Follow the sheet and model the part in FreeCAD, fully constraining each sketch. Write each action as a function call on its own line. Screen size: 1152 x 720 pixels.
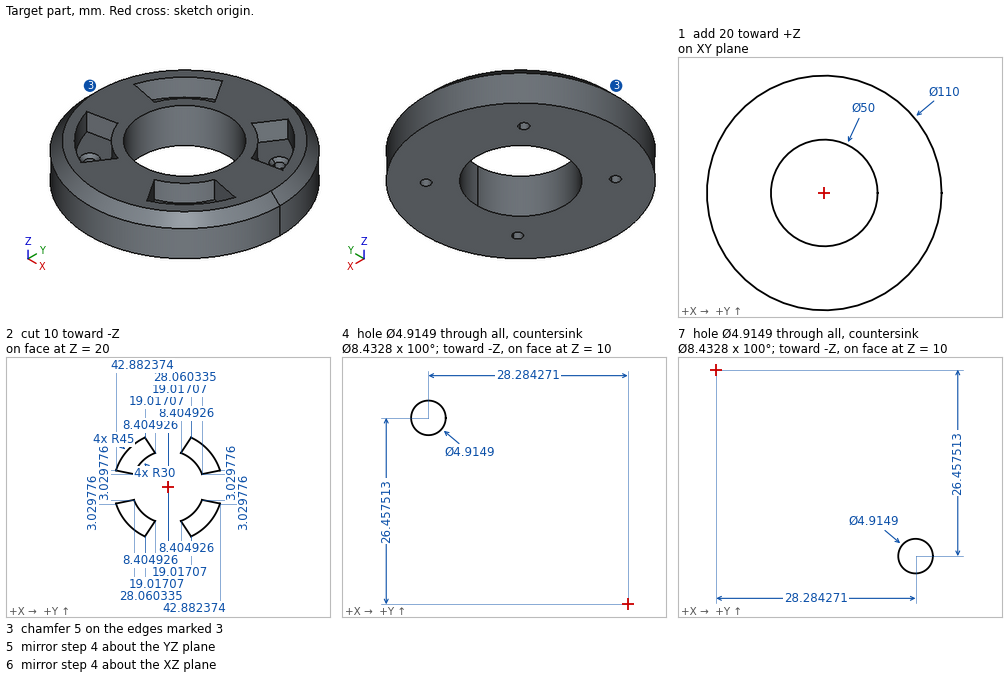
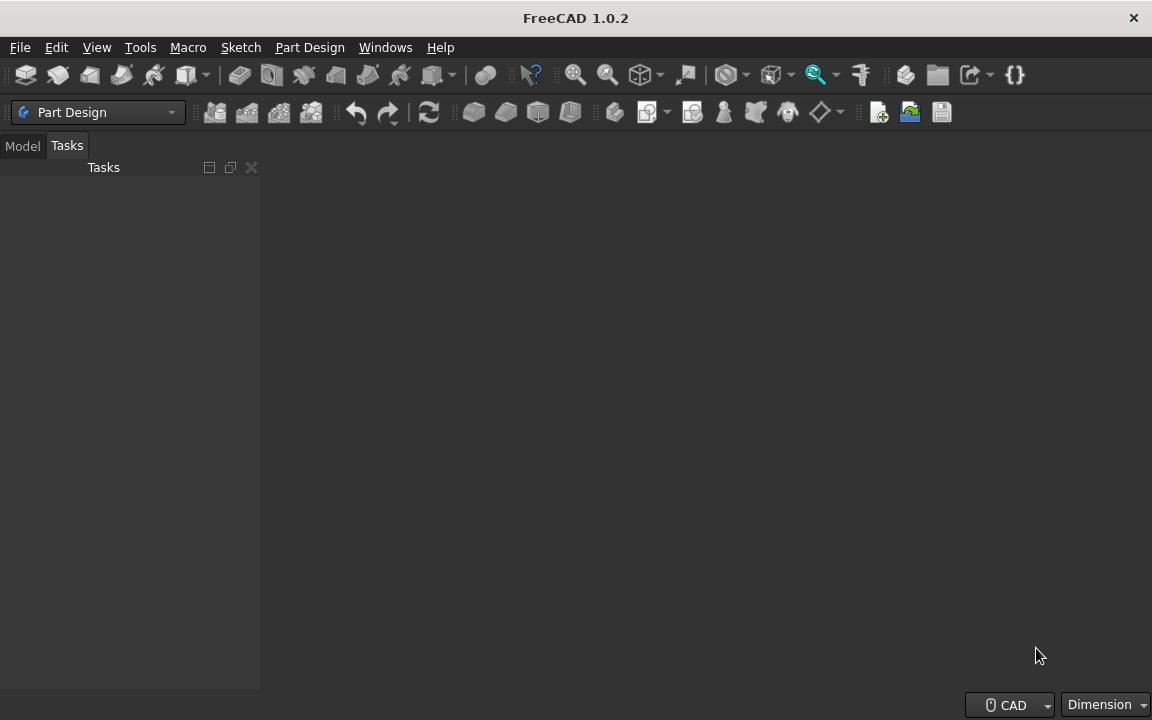
click(878, 112)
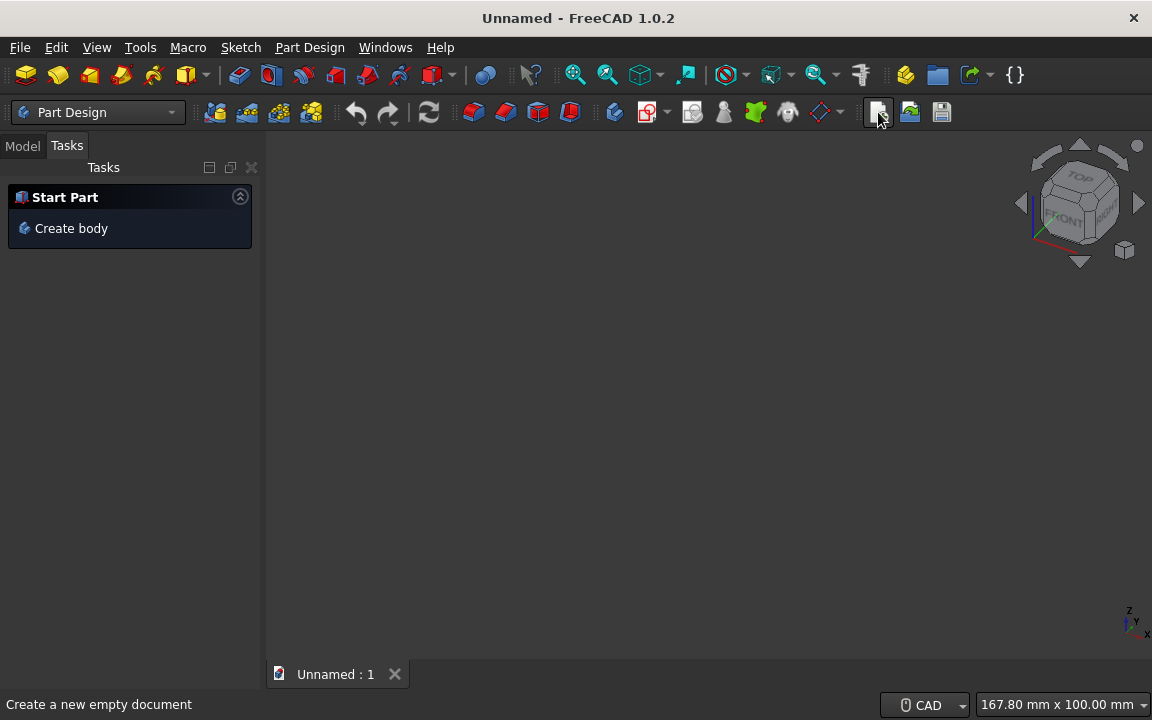
click(648, 112)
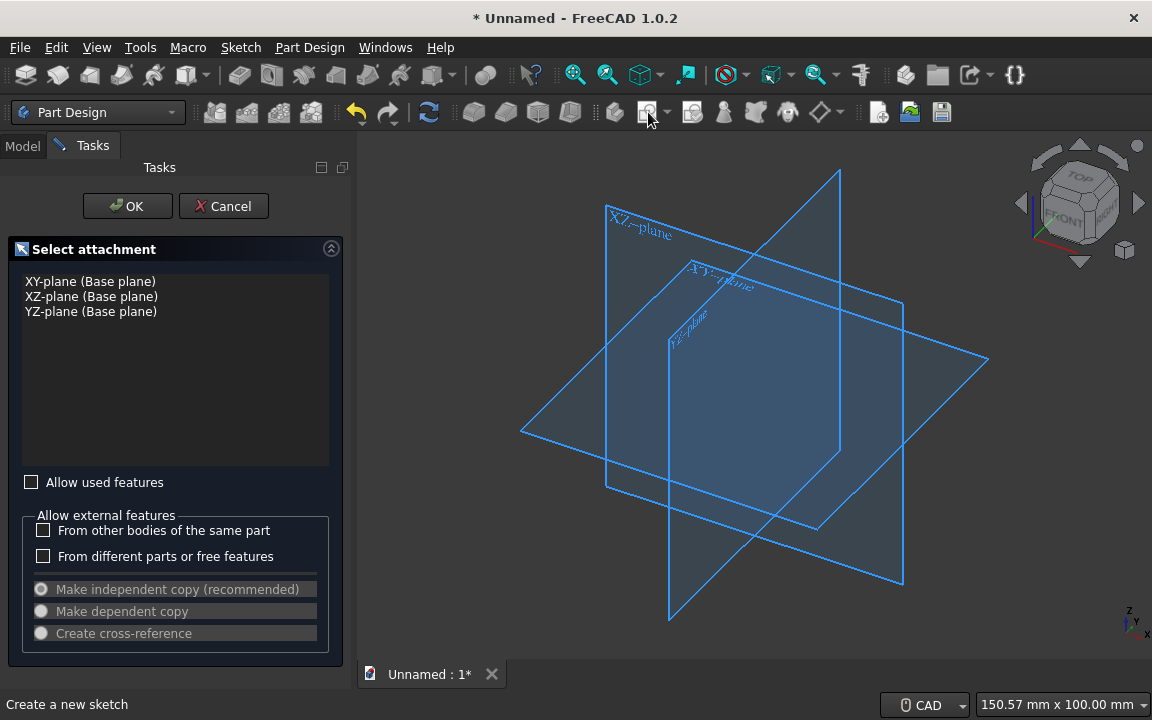
click(82, 282)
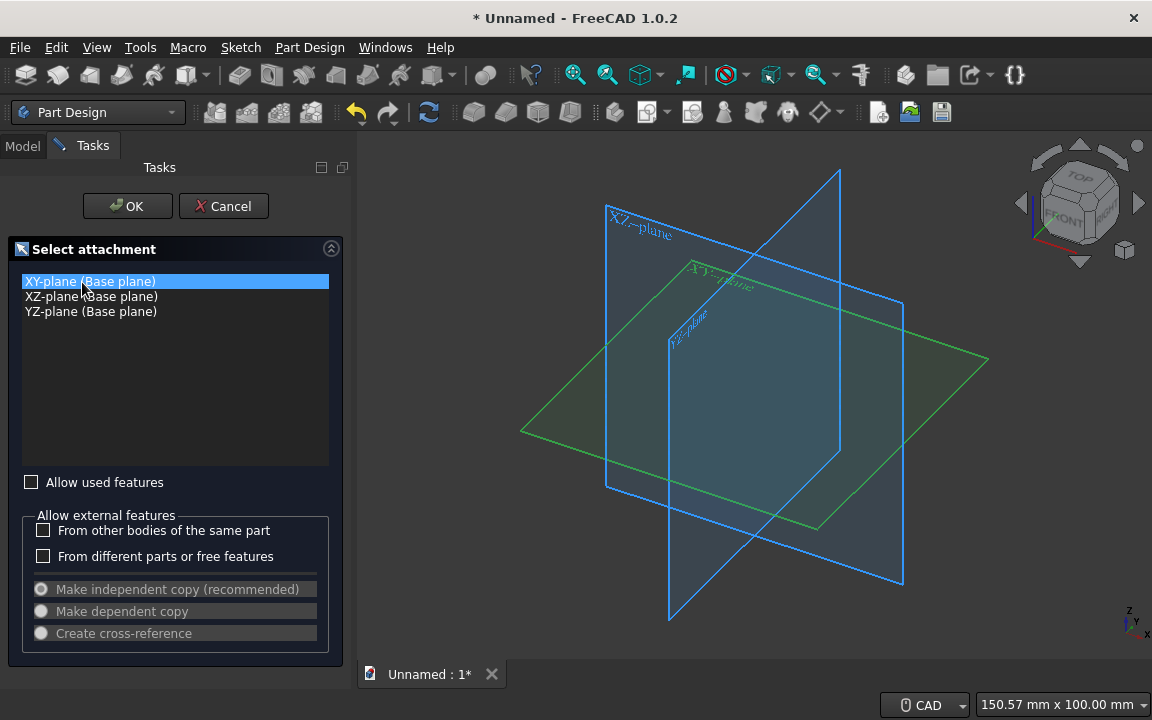
click(128, 206)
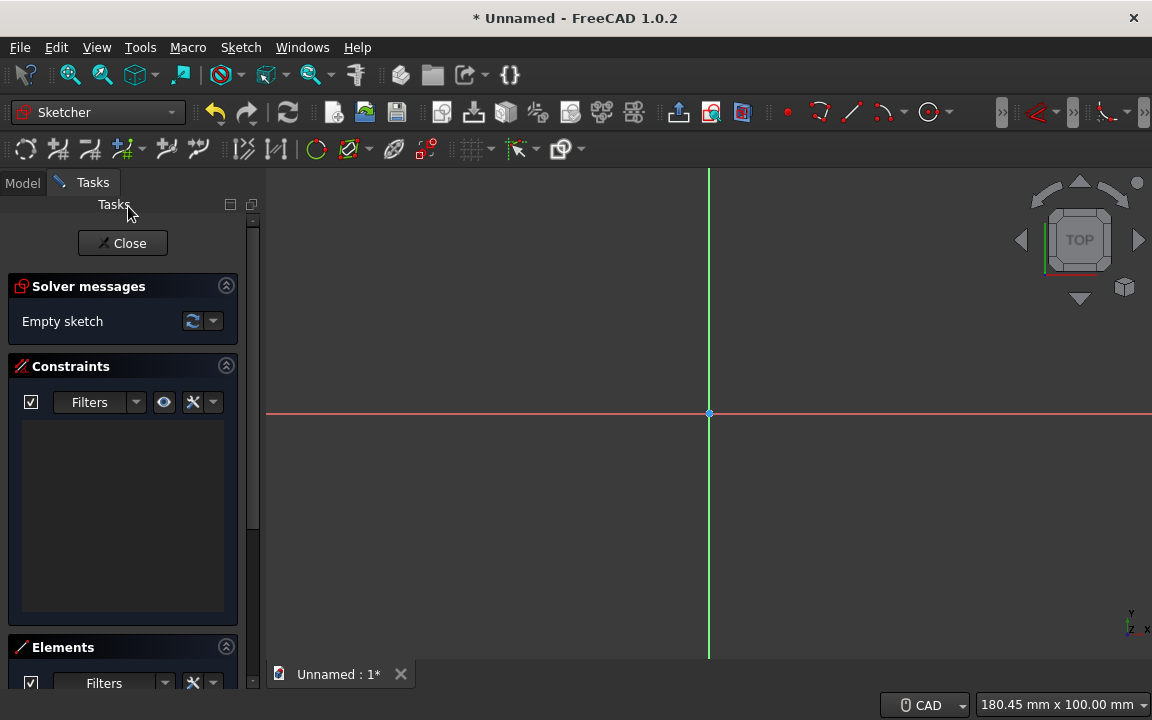
scroll(557, 414, down, 3)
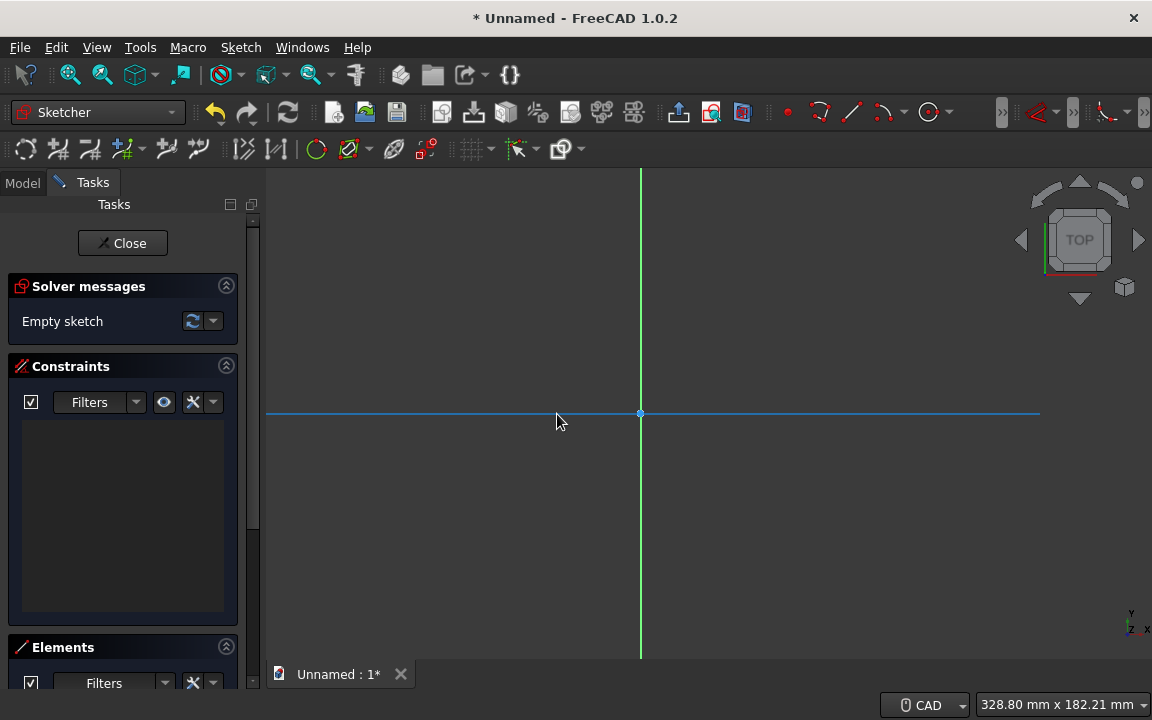
click(930, 112)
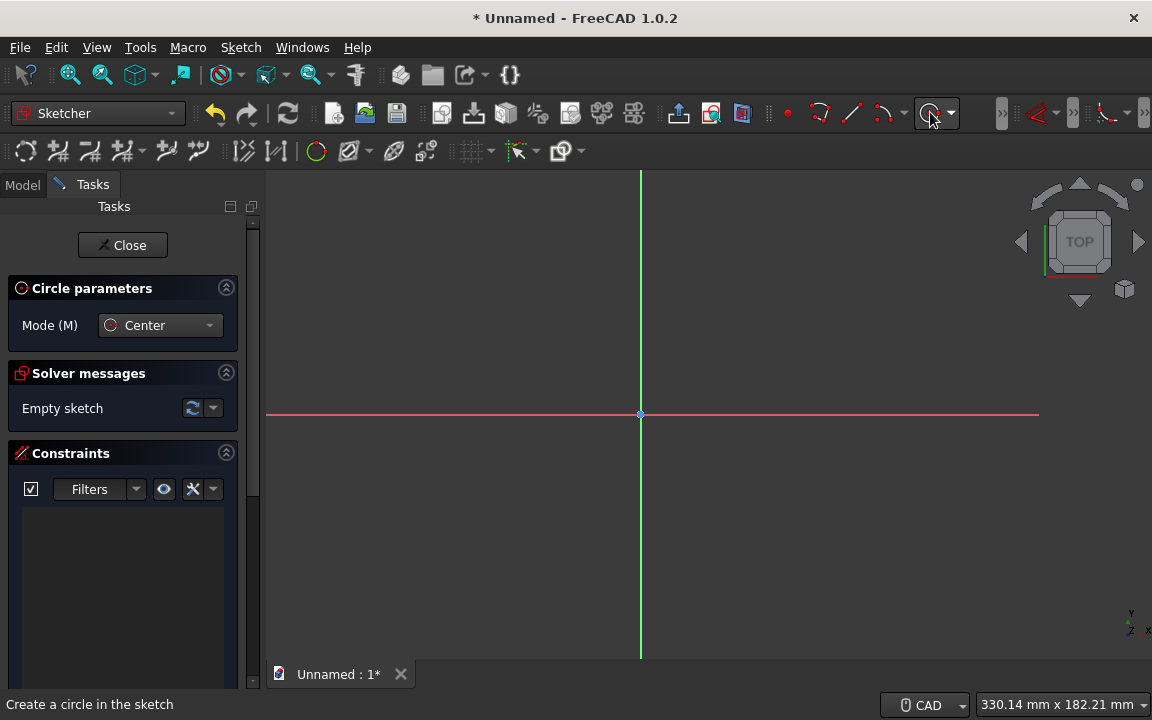
click(641, 415)
click(745, 311)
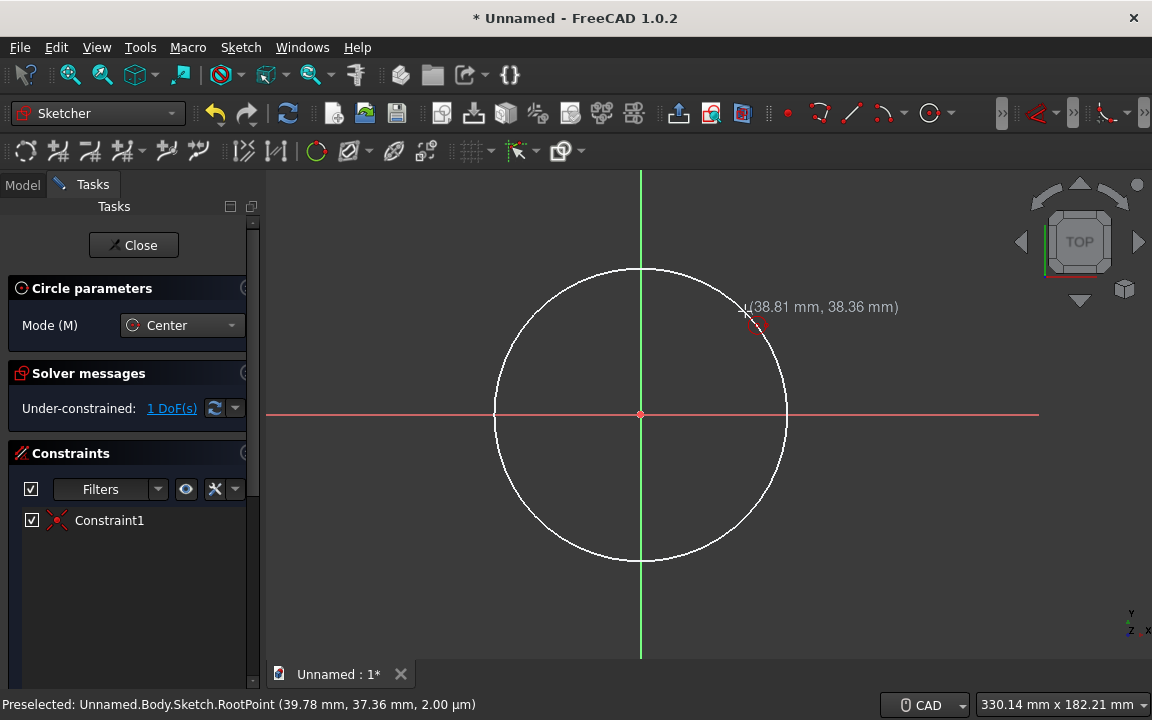
click(641, 415)
click(688, 368)
key(Escape)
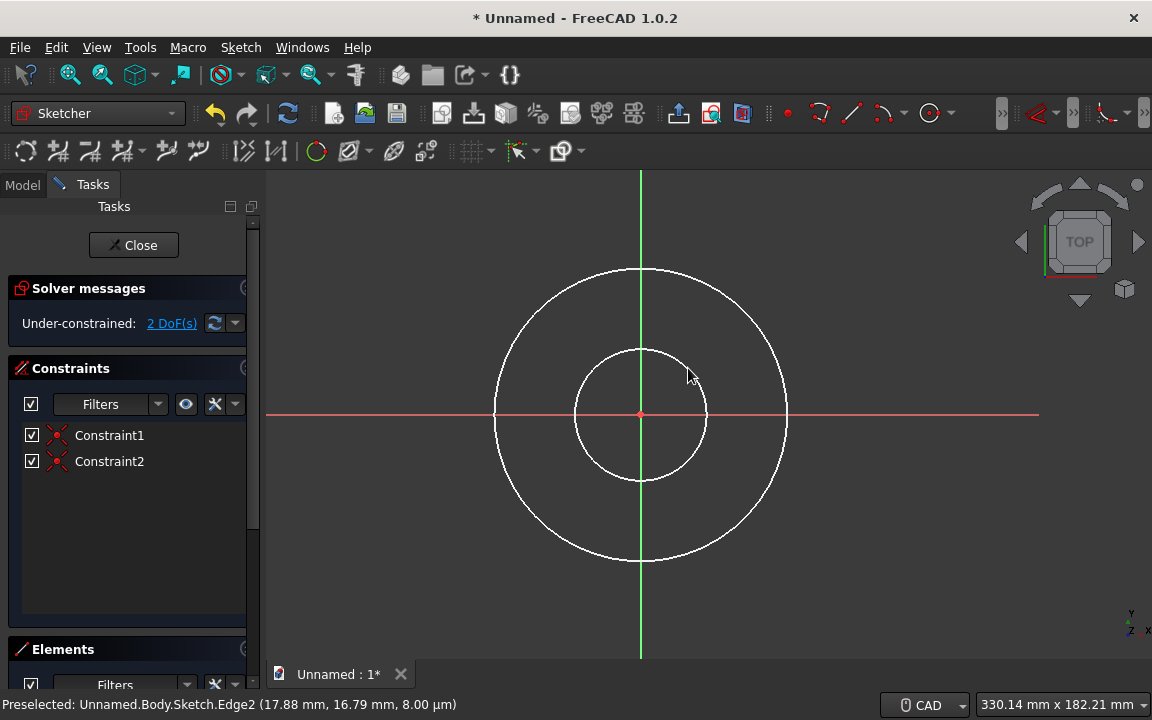
click(1036, 114)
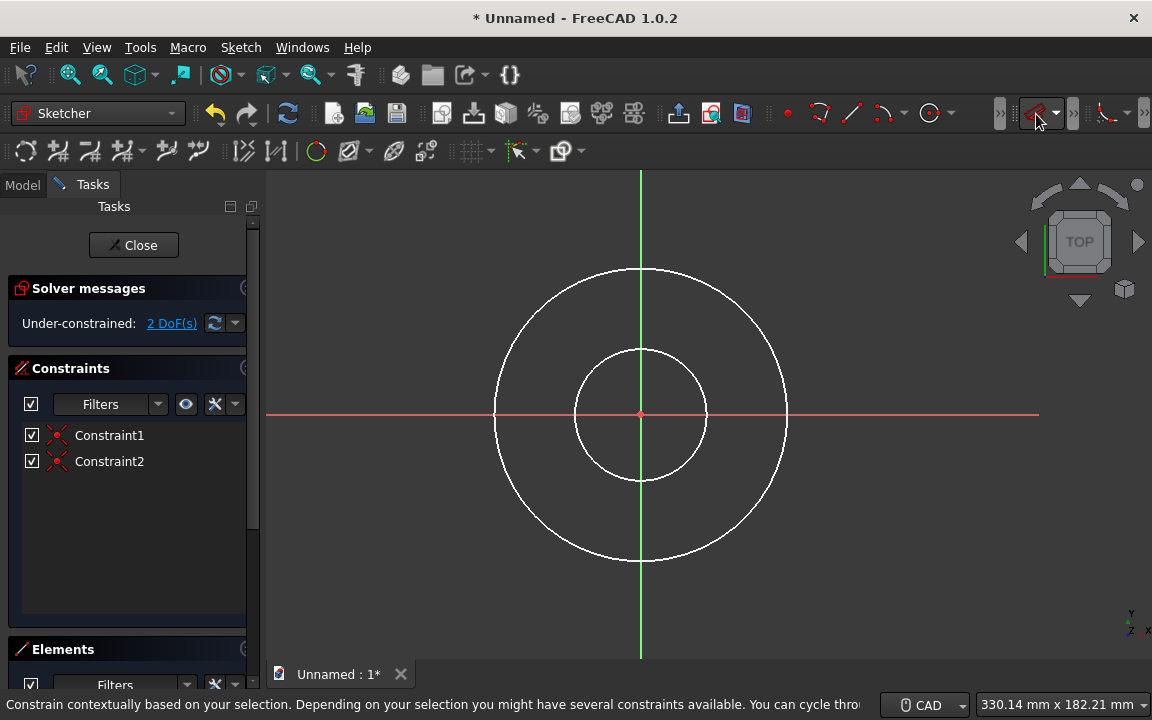
click(744, 311)
click(767, 288)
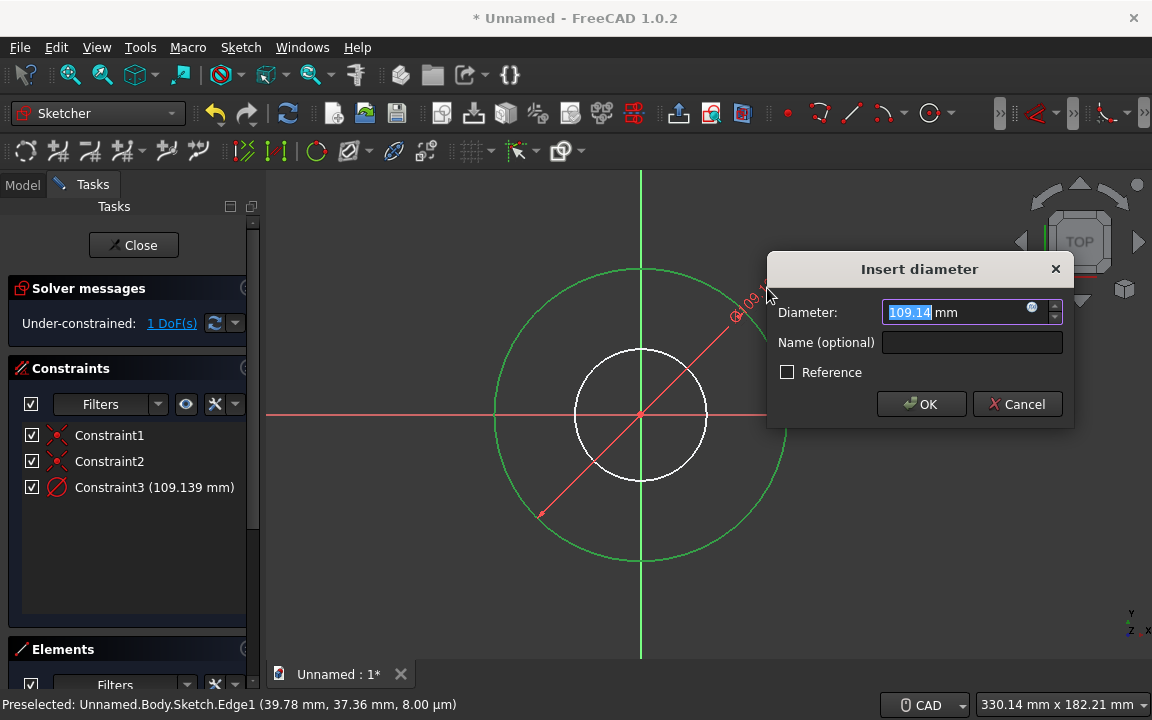
text(110)
key(Return)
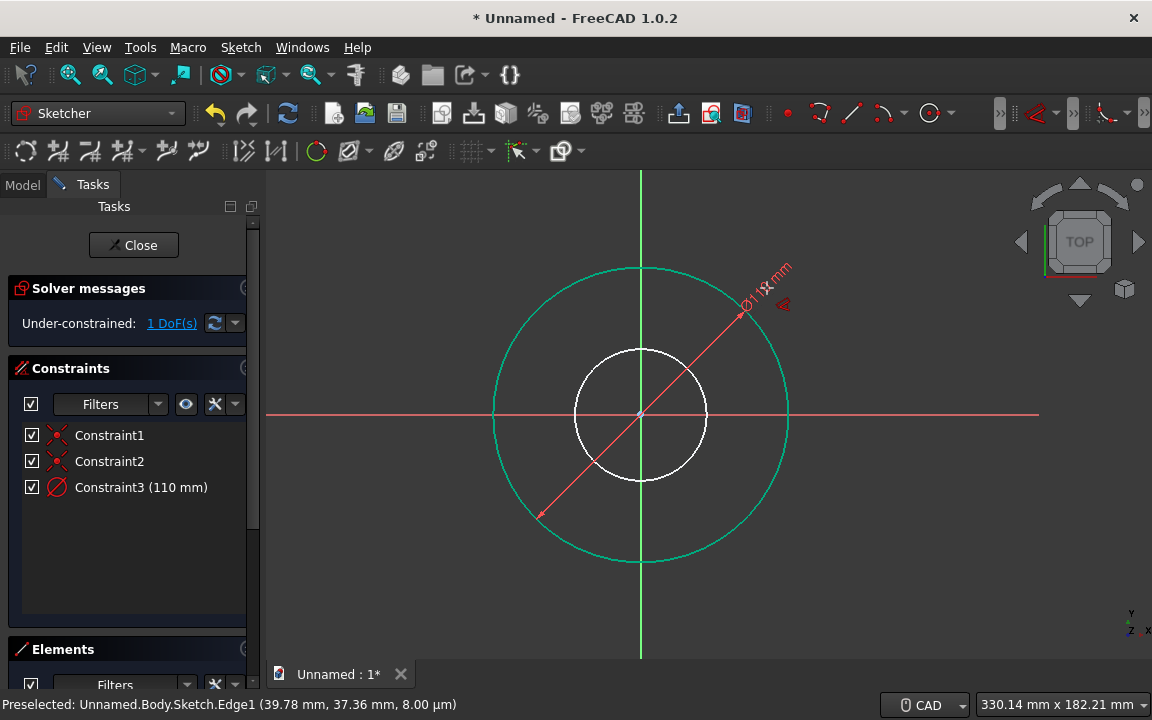
click(687, 368)
click(709, 345)